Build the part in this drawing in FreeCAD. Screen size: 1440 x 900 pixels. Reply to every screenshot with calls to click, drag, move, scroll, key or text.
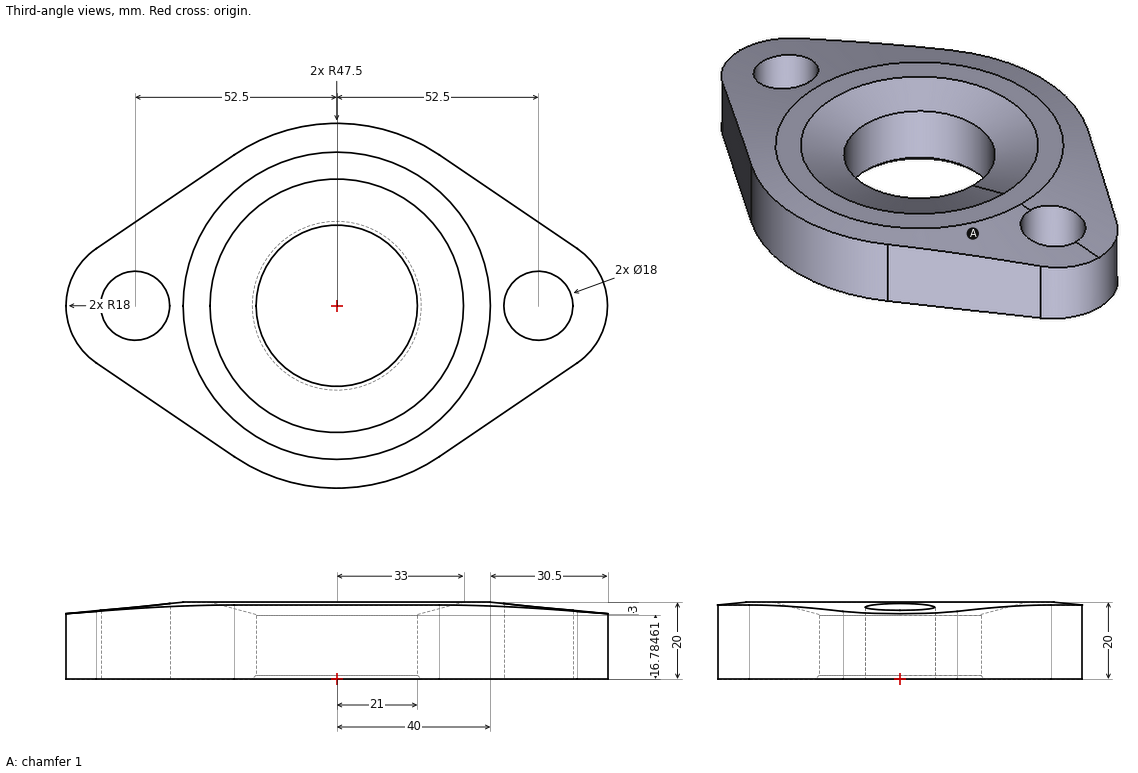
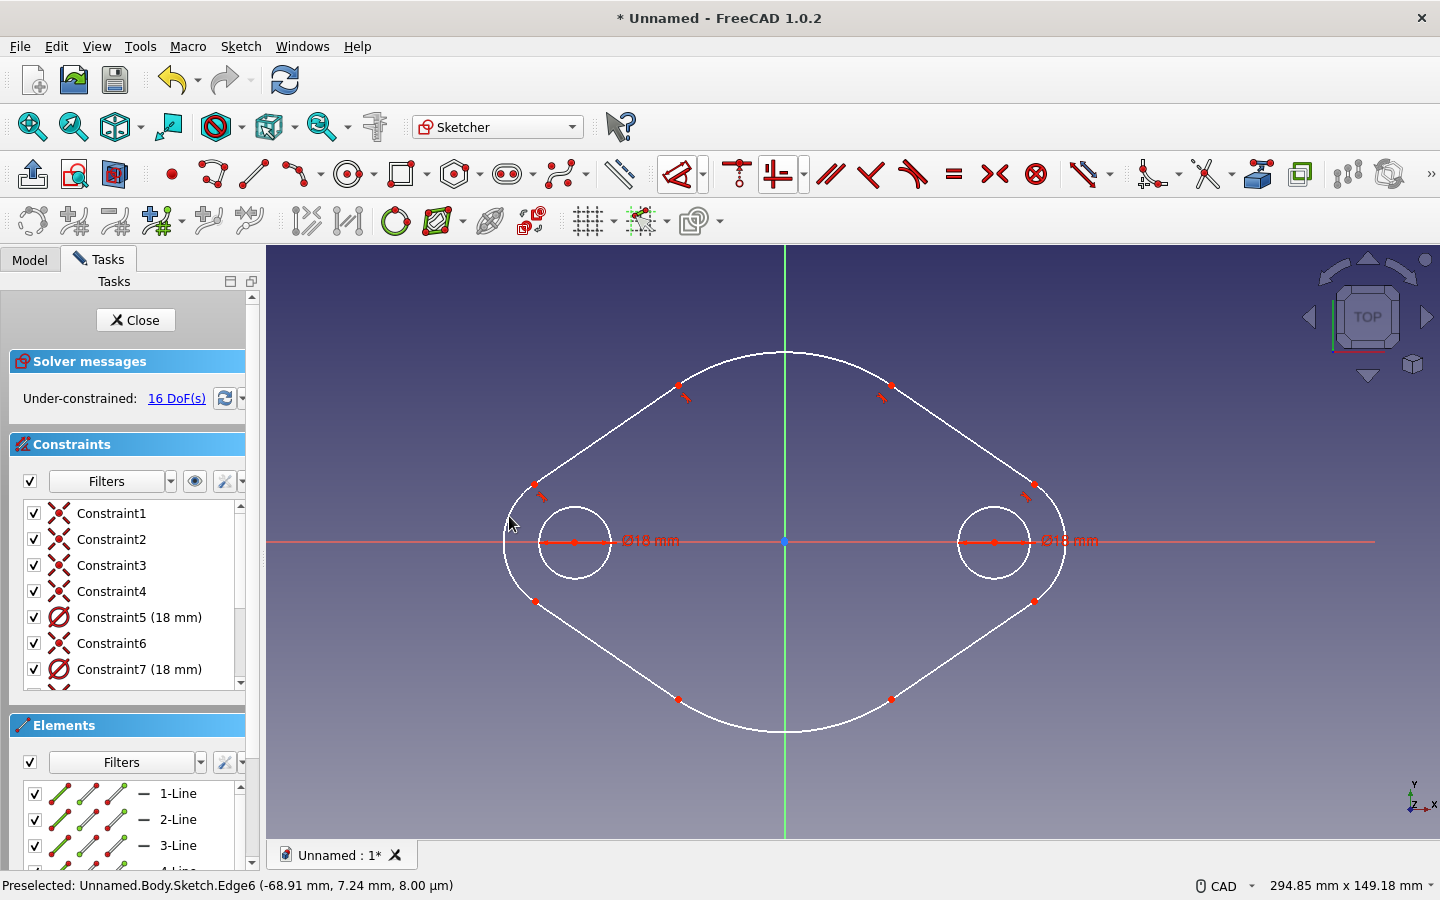
click(578, 631)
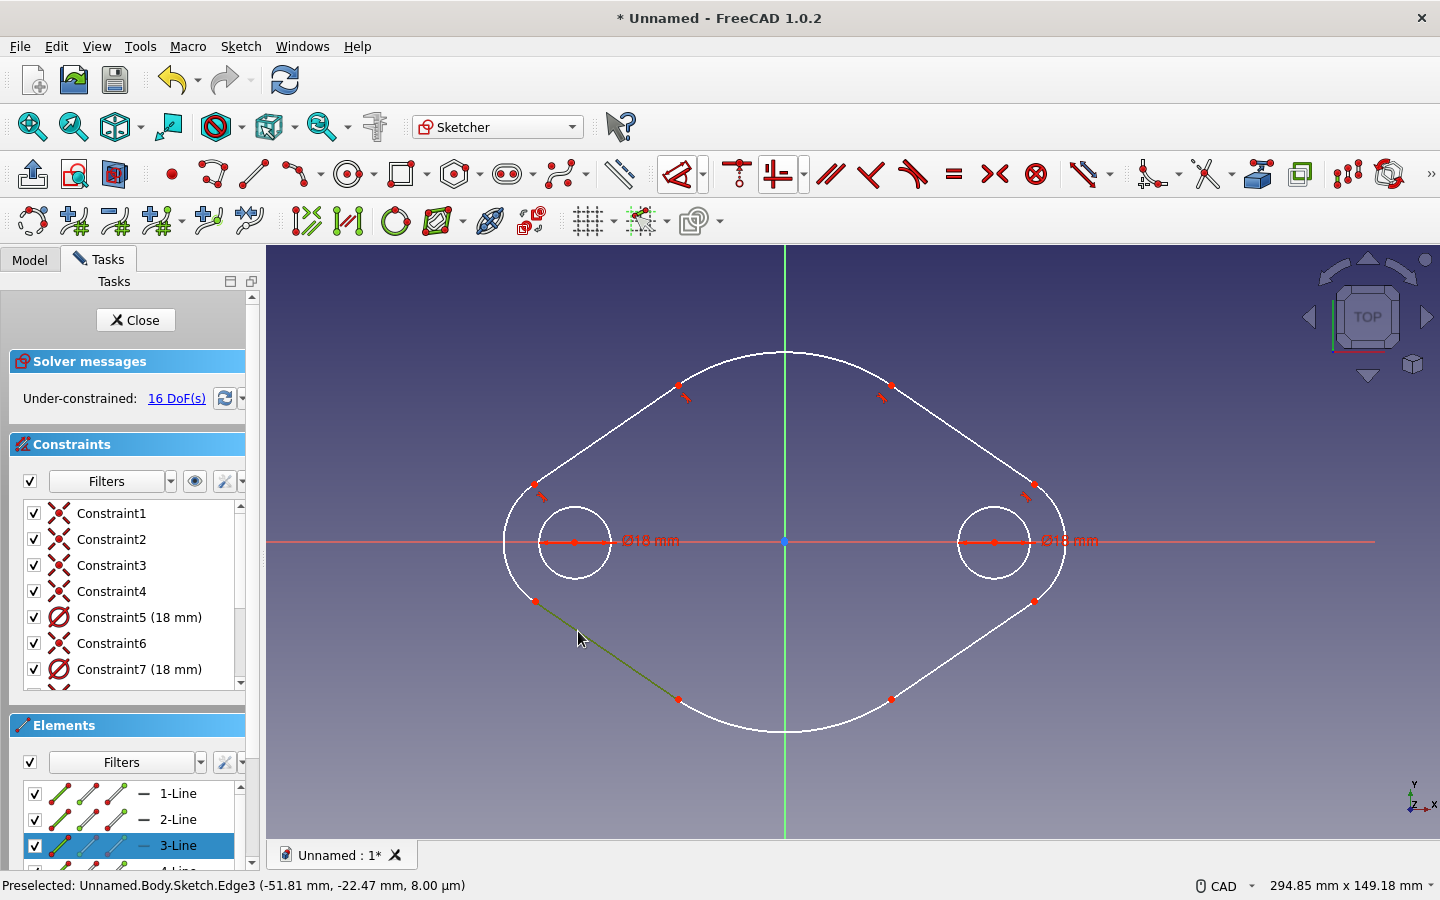
click(509, 516)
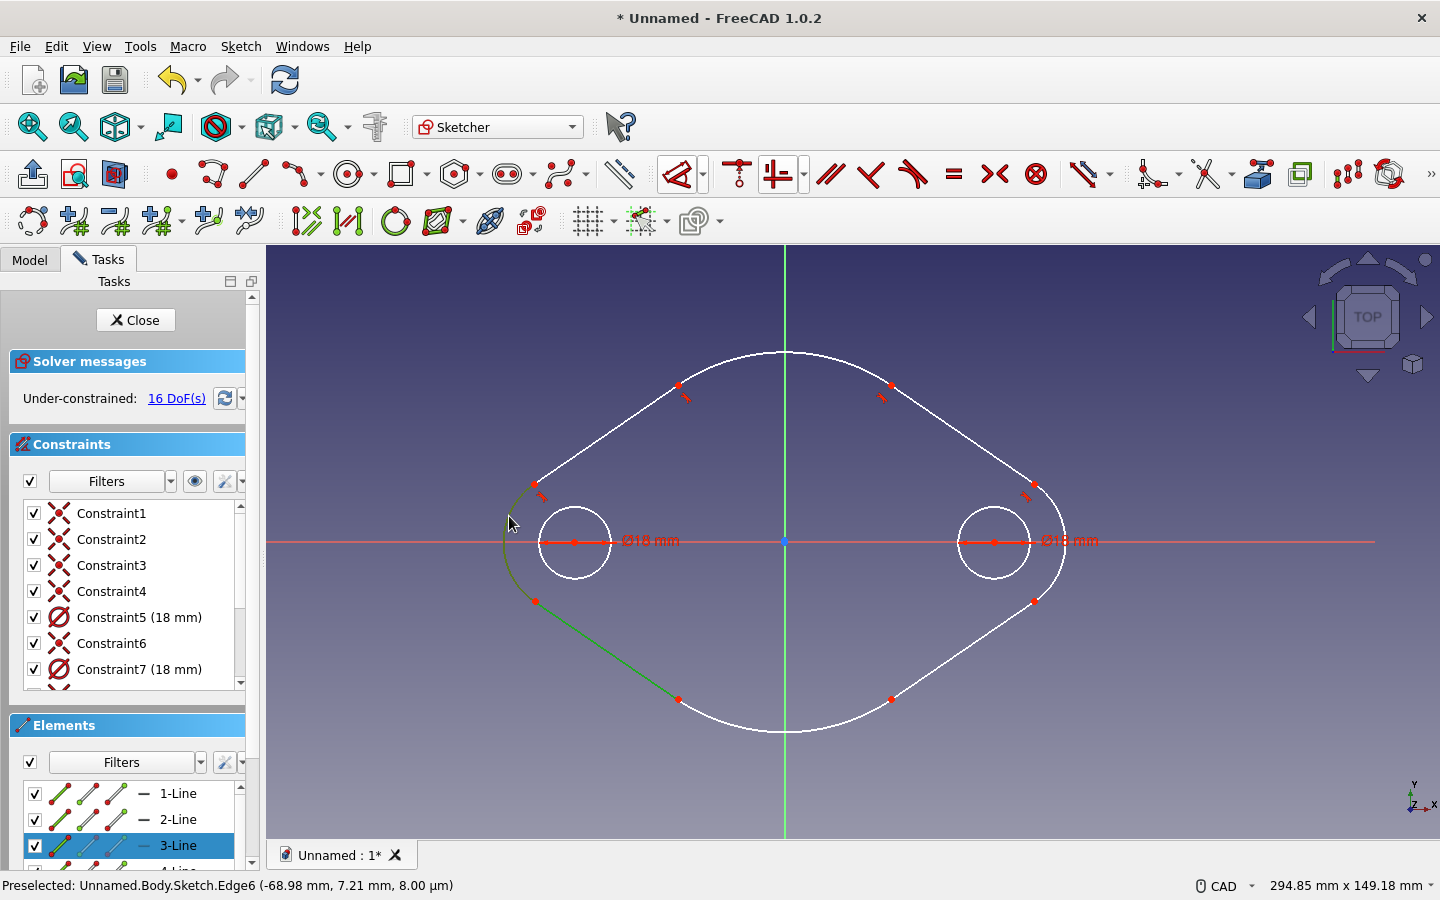
key(t)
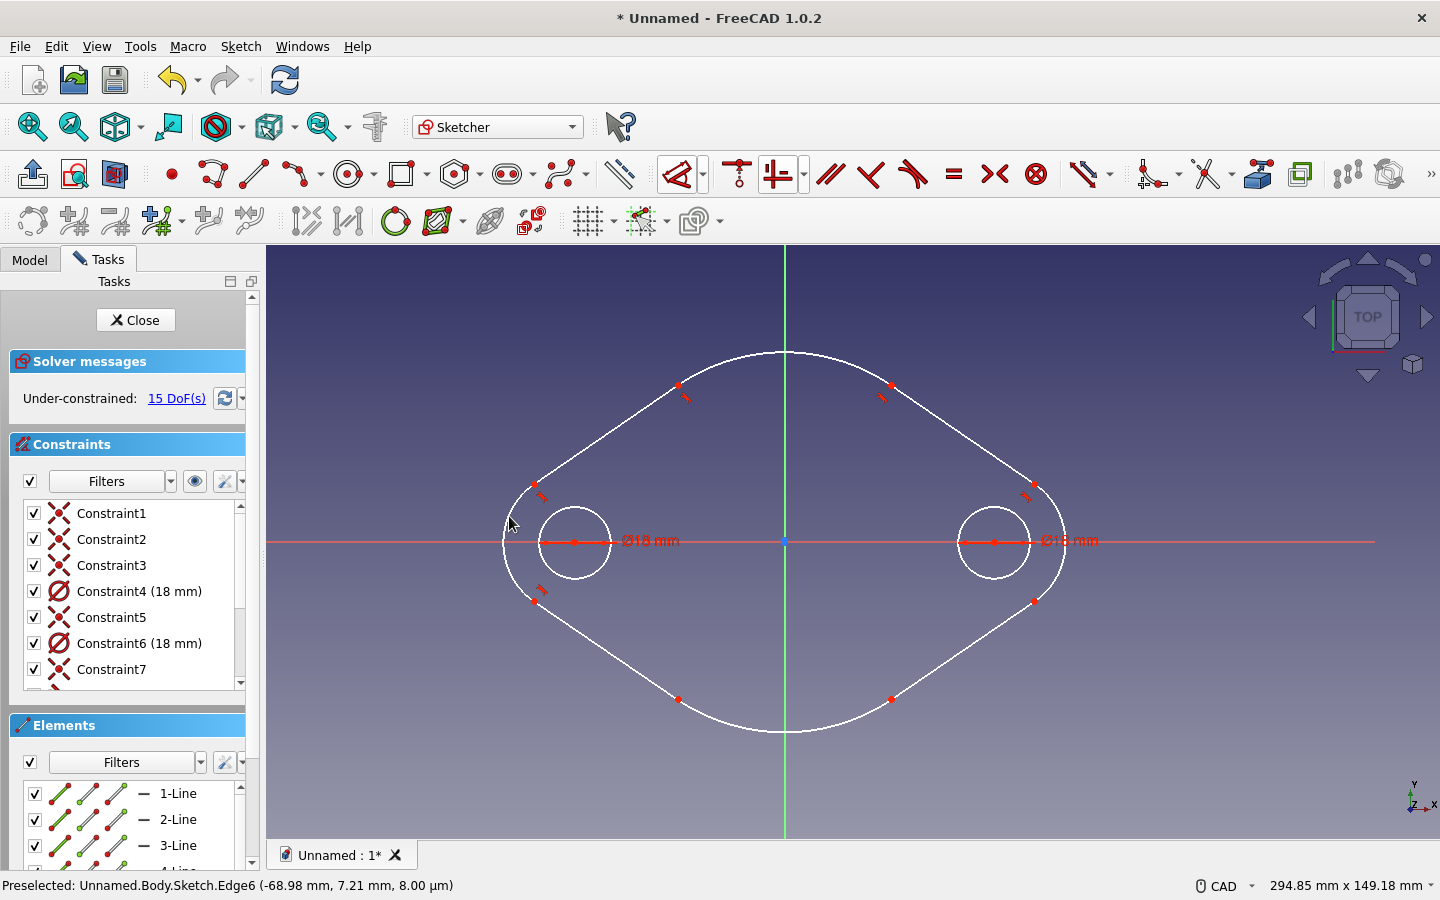
click(578, 631)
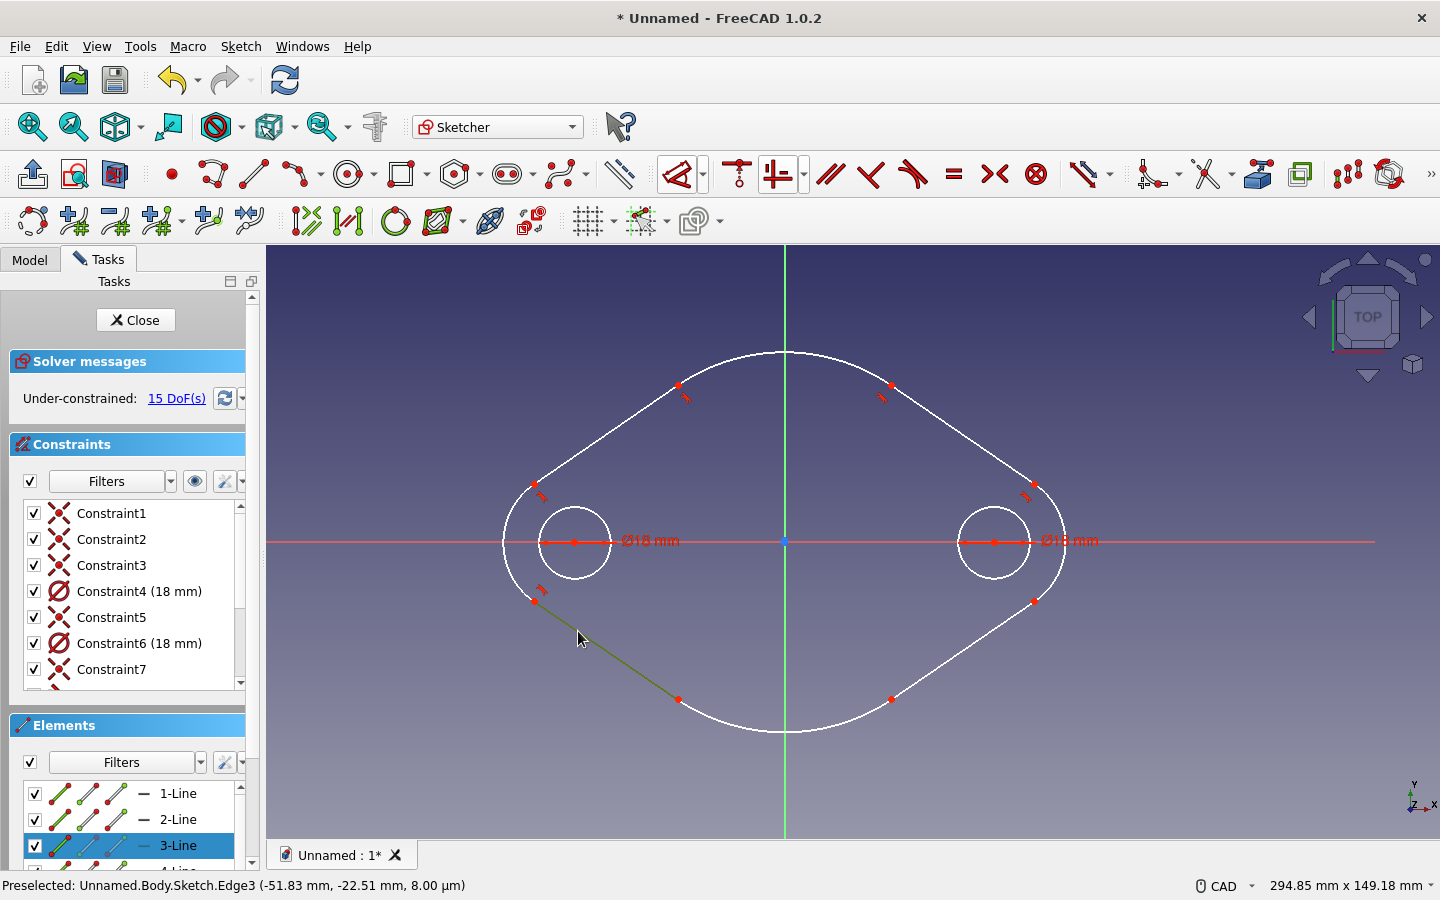
click(740, 727)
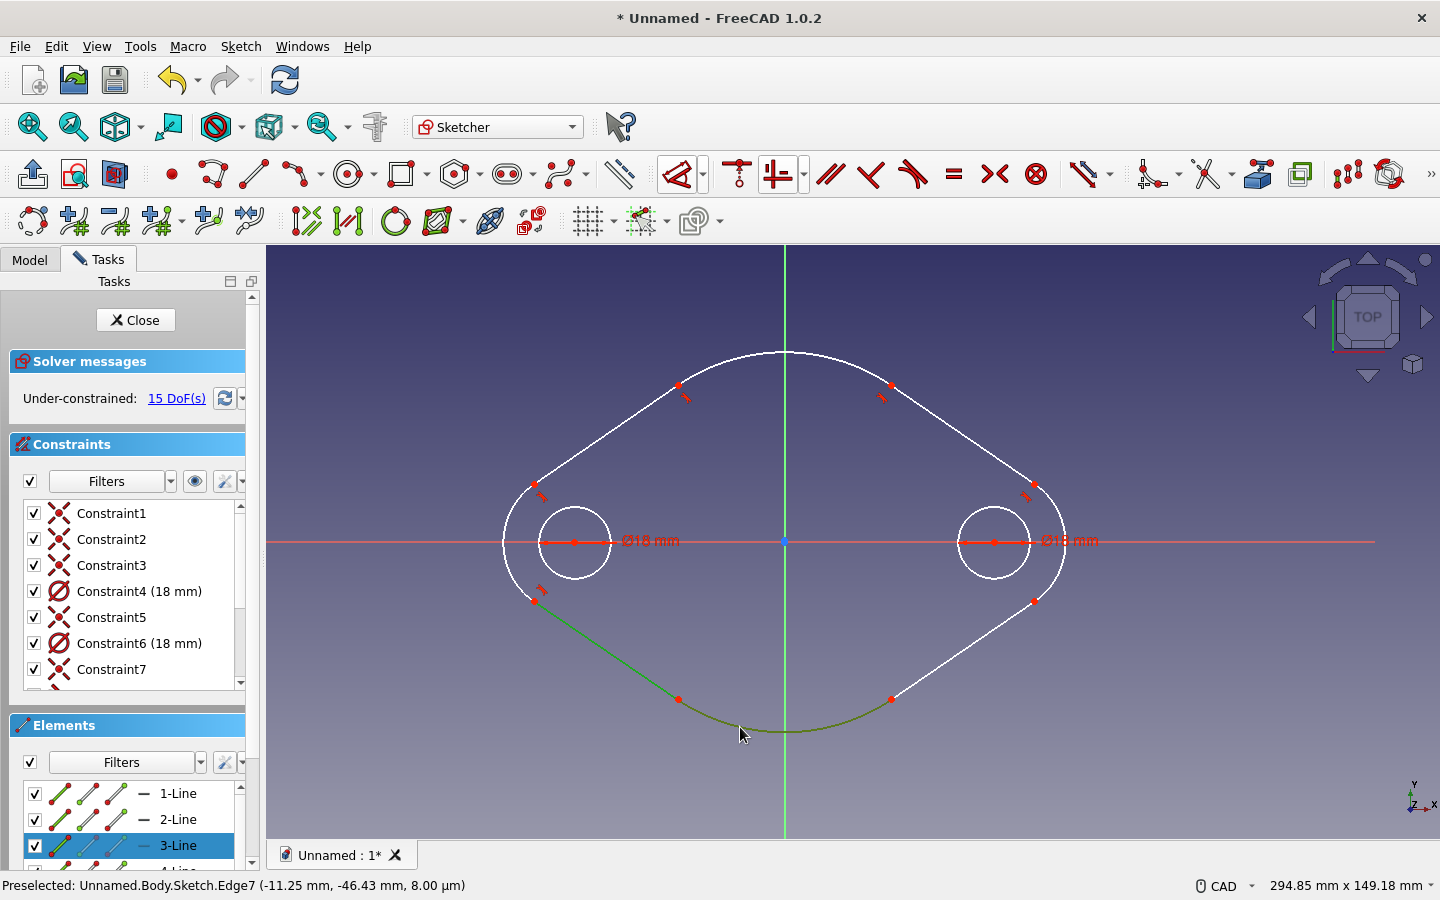
key(t)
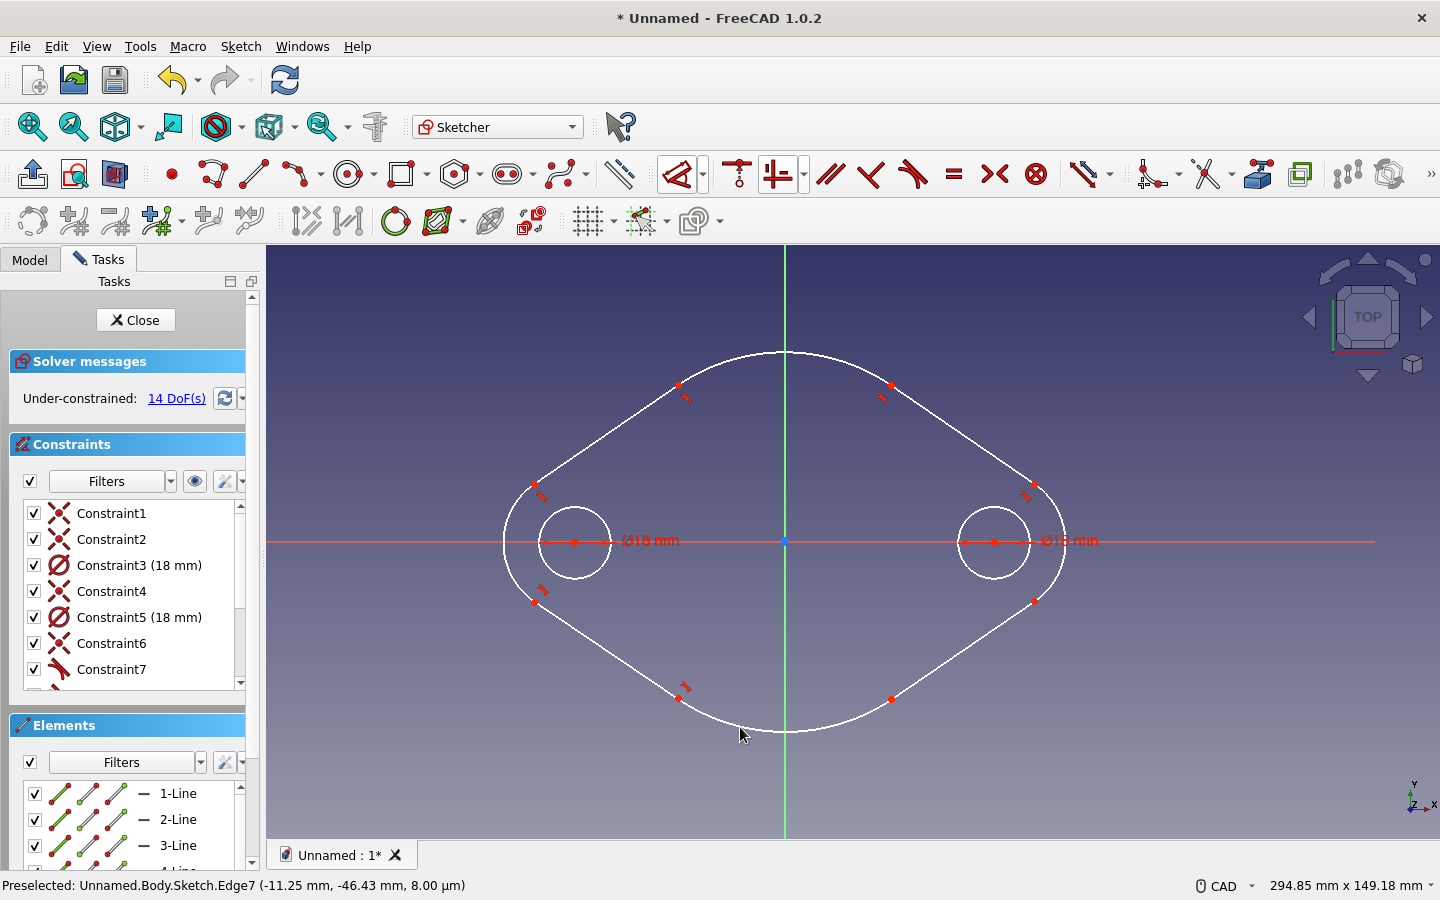
click(934, 671)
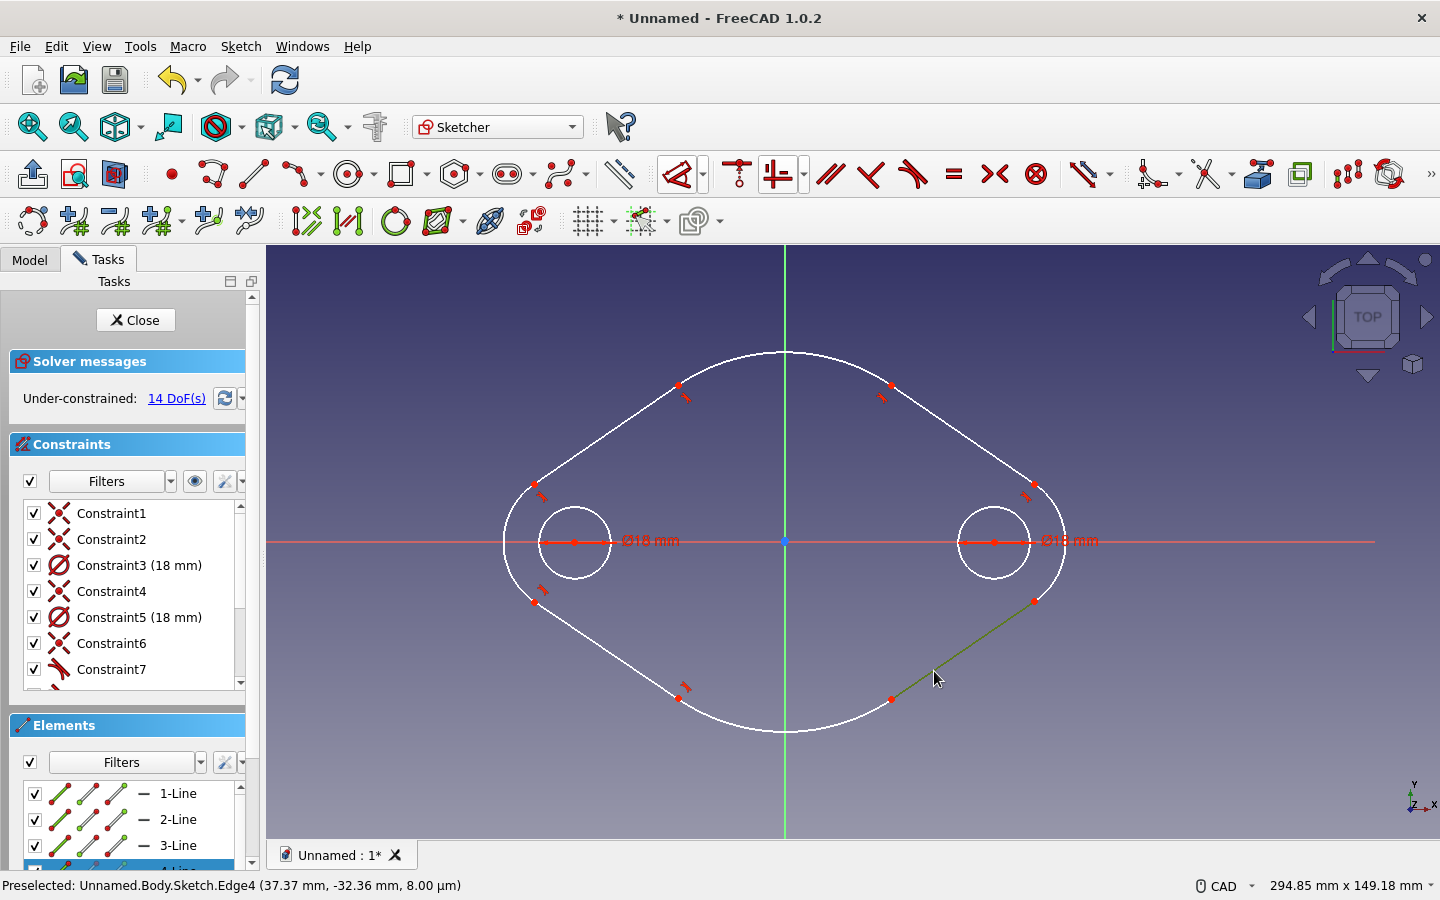
click(740, 726)